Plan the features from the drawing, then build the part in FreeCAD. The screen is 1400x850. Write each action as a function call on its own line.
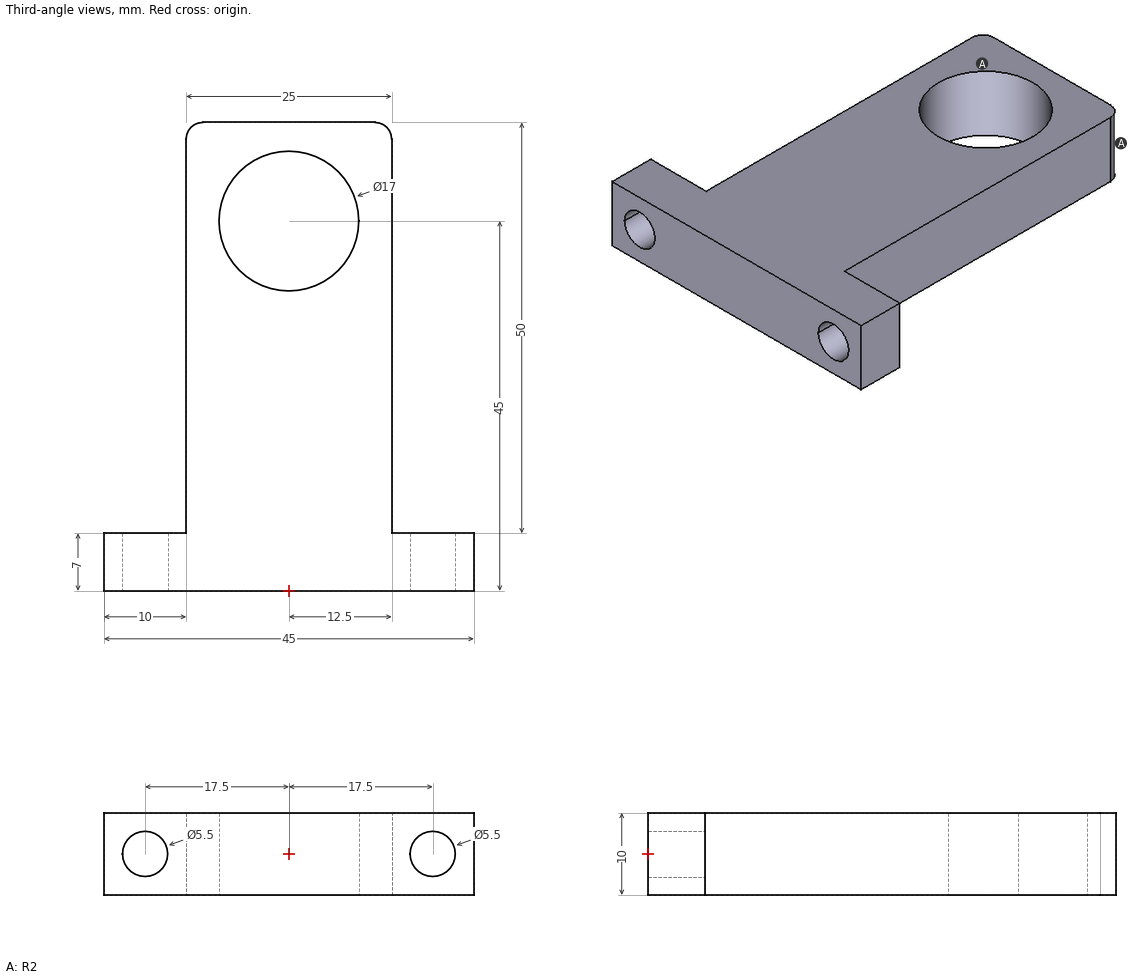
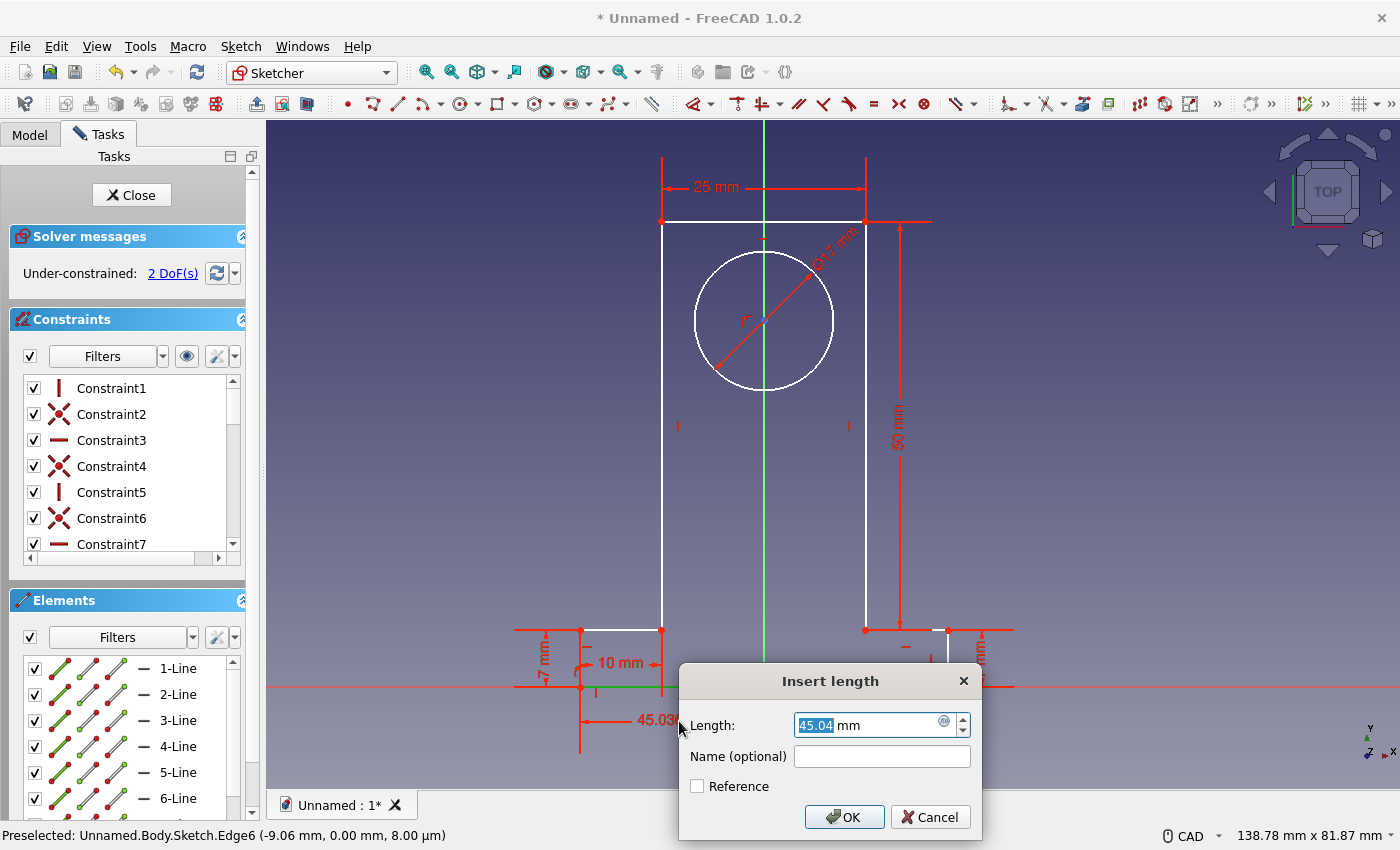
text(45)
key(Return)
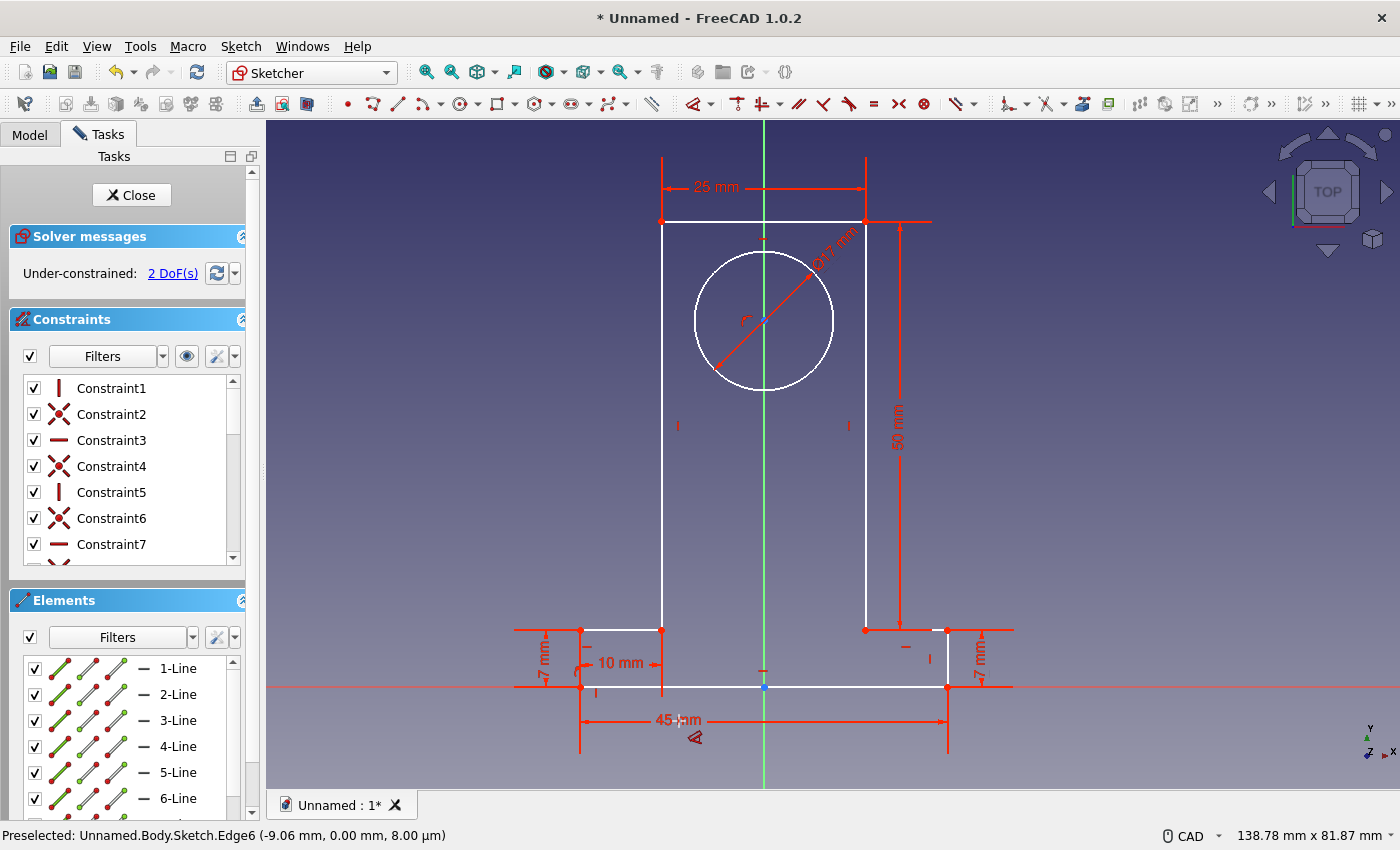
click(764, 321)
click(798, 504)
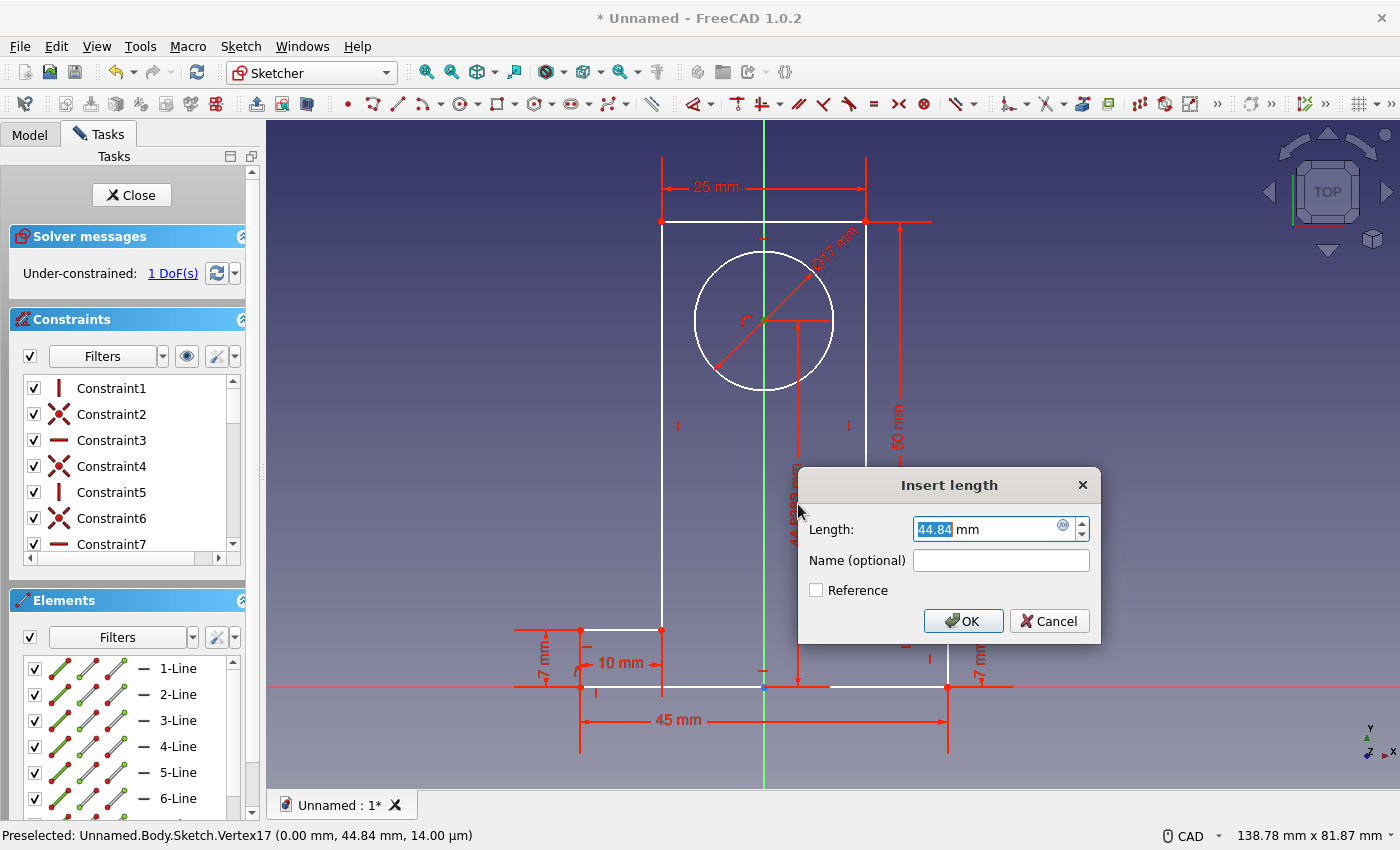
text(45)
key(Return)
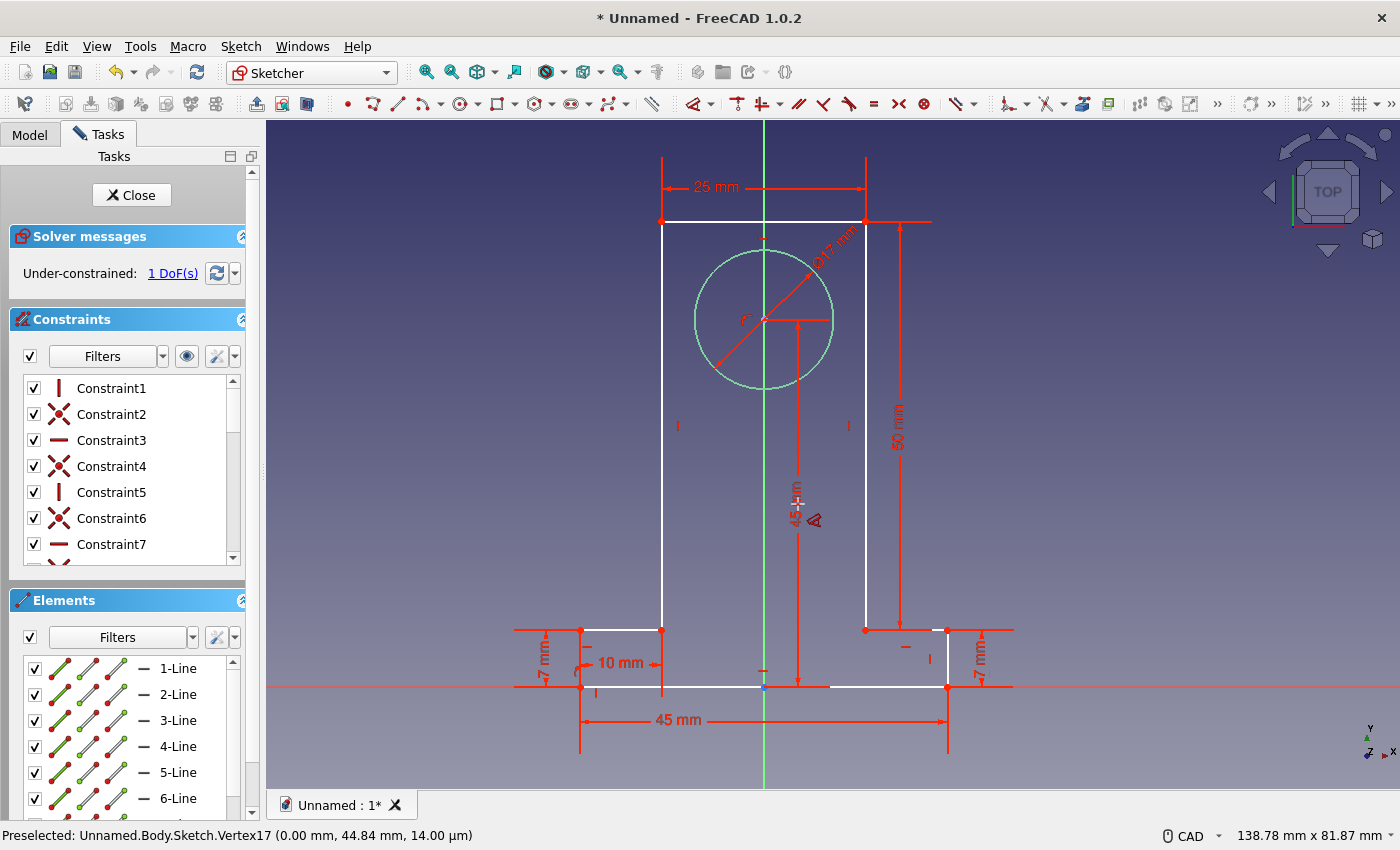
click(866, 630)
click(815, 721)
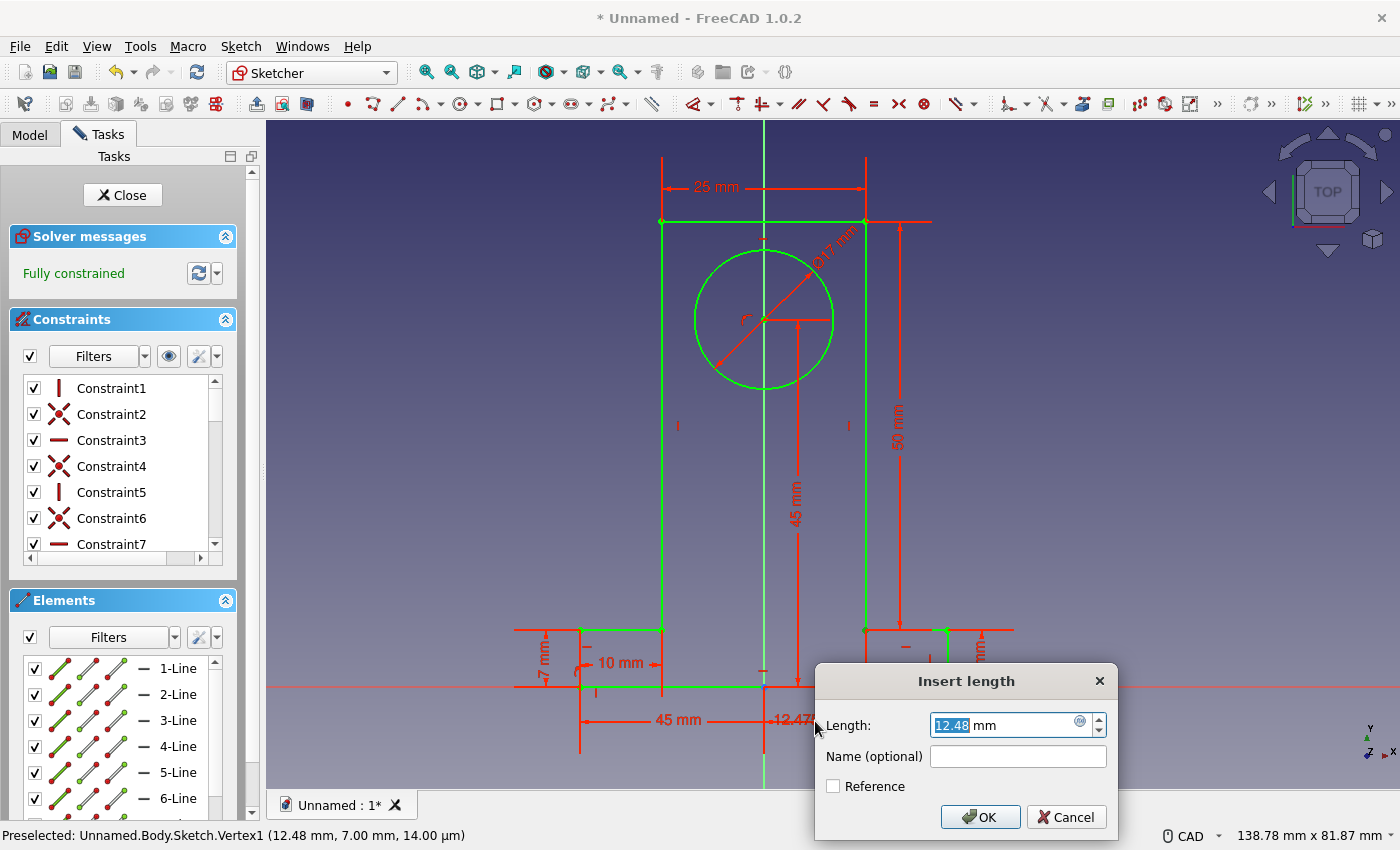
text(12.5)
key(Return)
key(Escape)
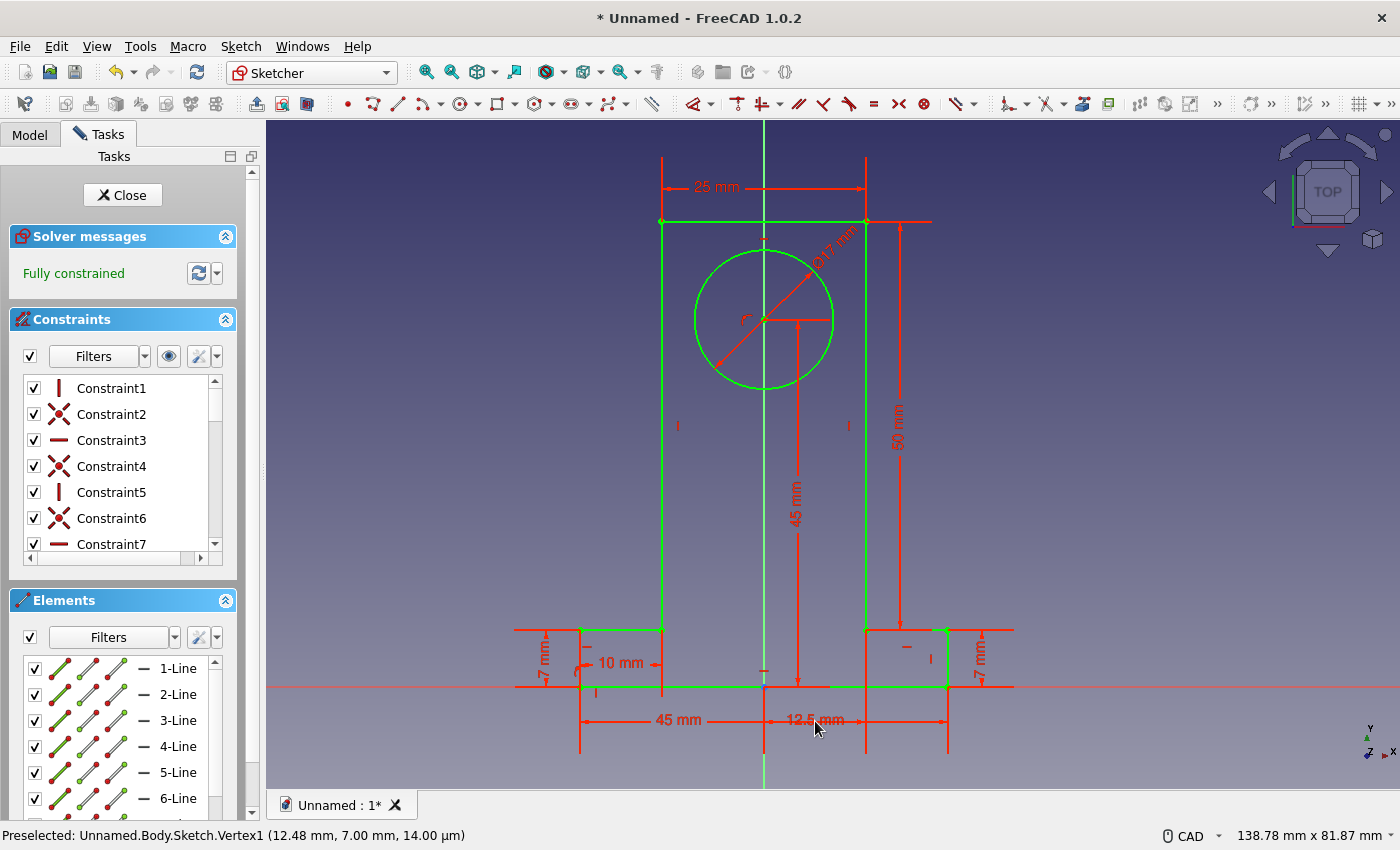
click(123, 195)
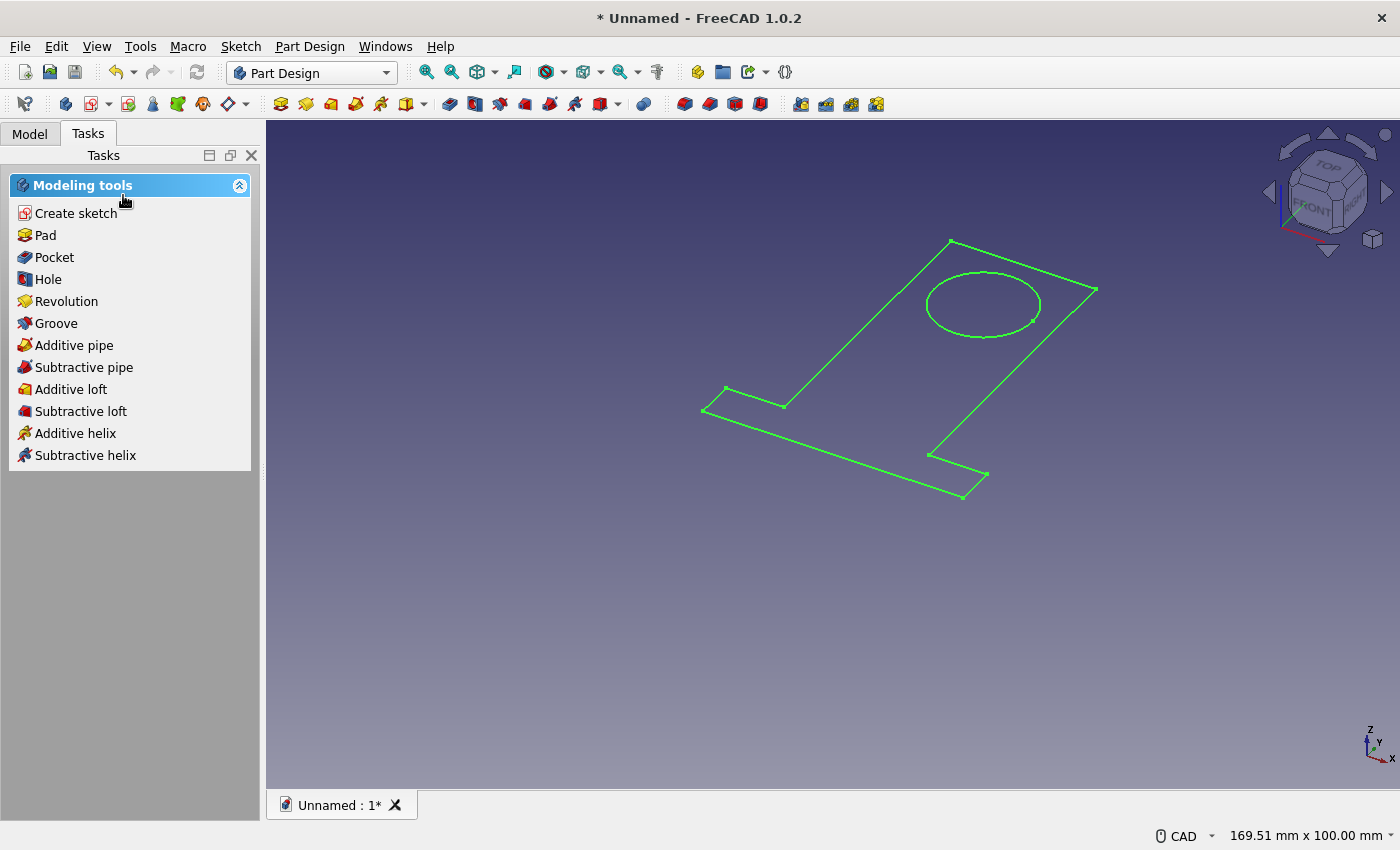
click(281, 104)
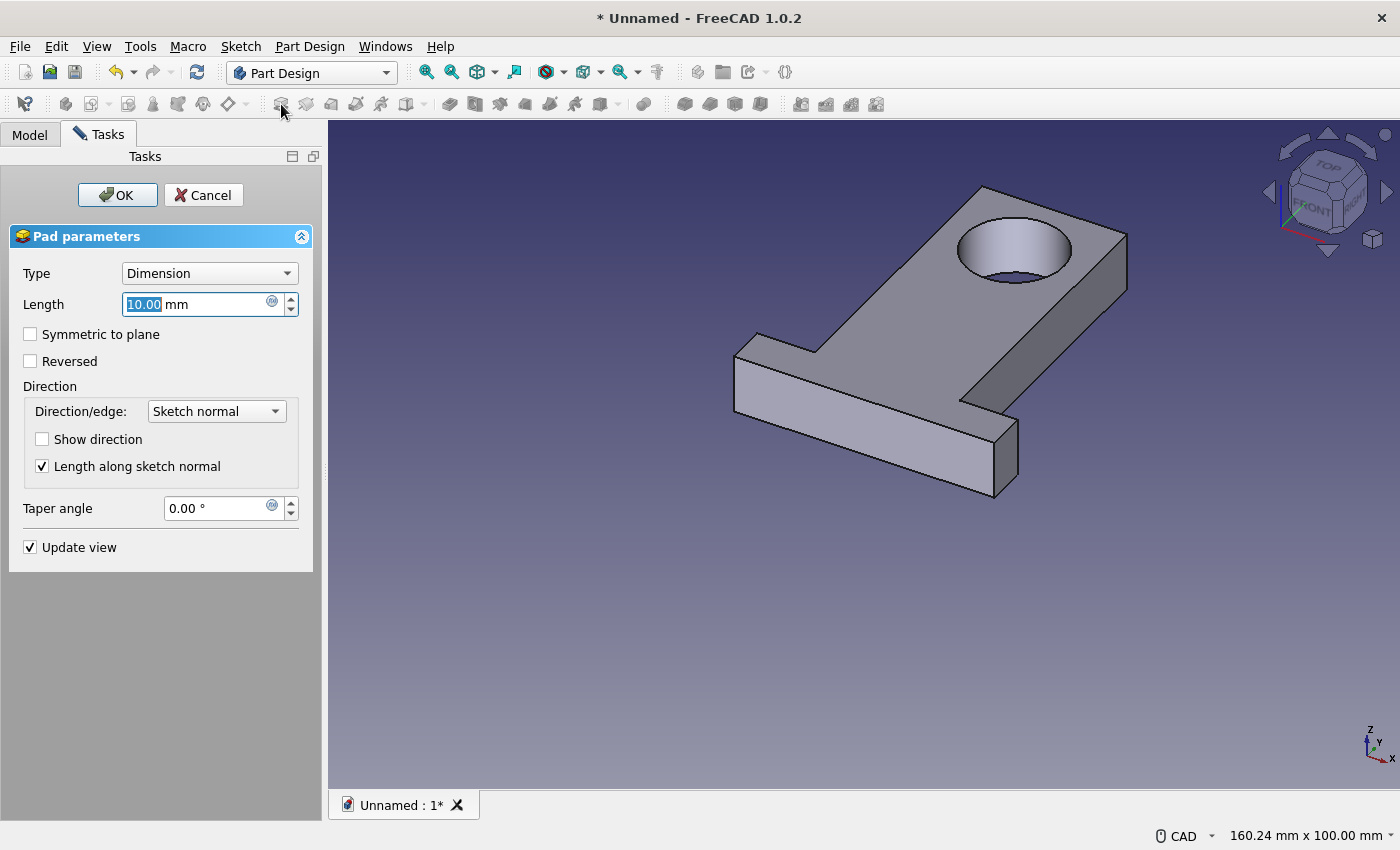
text(10)
key(Tab)